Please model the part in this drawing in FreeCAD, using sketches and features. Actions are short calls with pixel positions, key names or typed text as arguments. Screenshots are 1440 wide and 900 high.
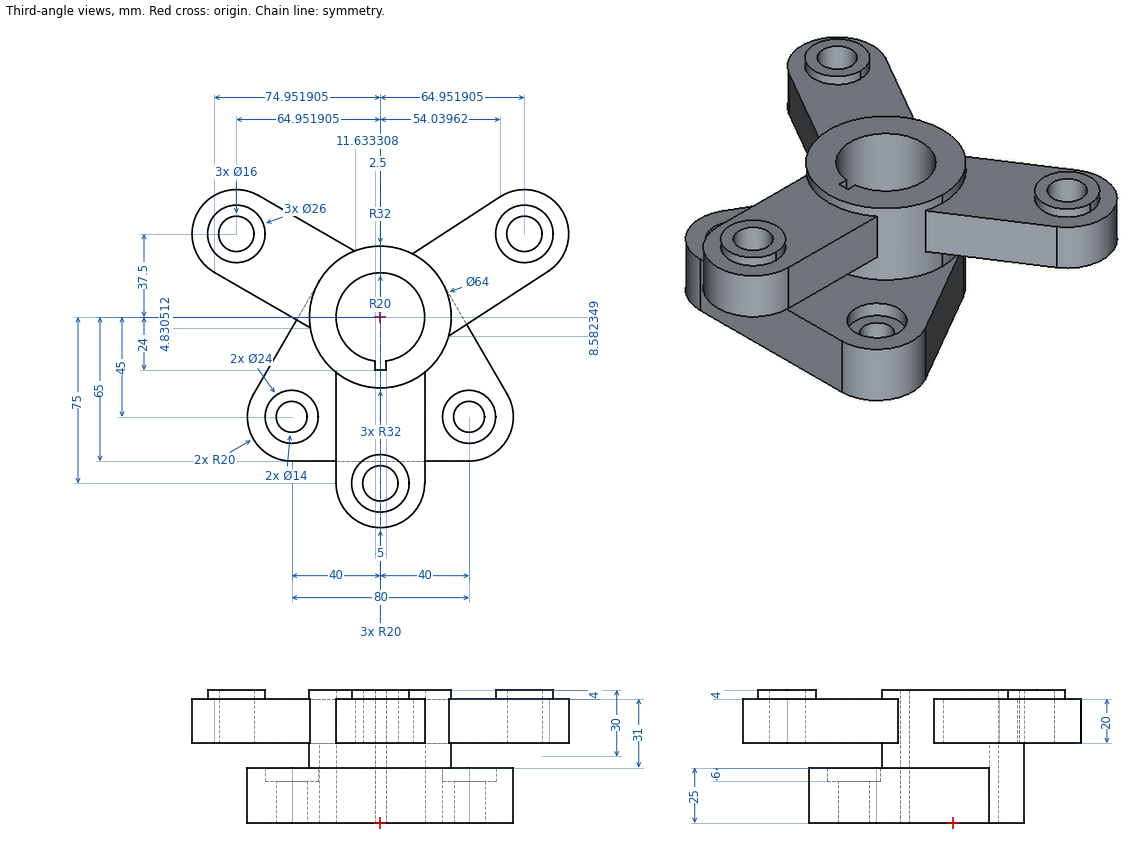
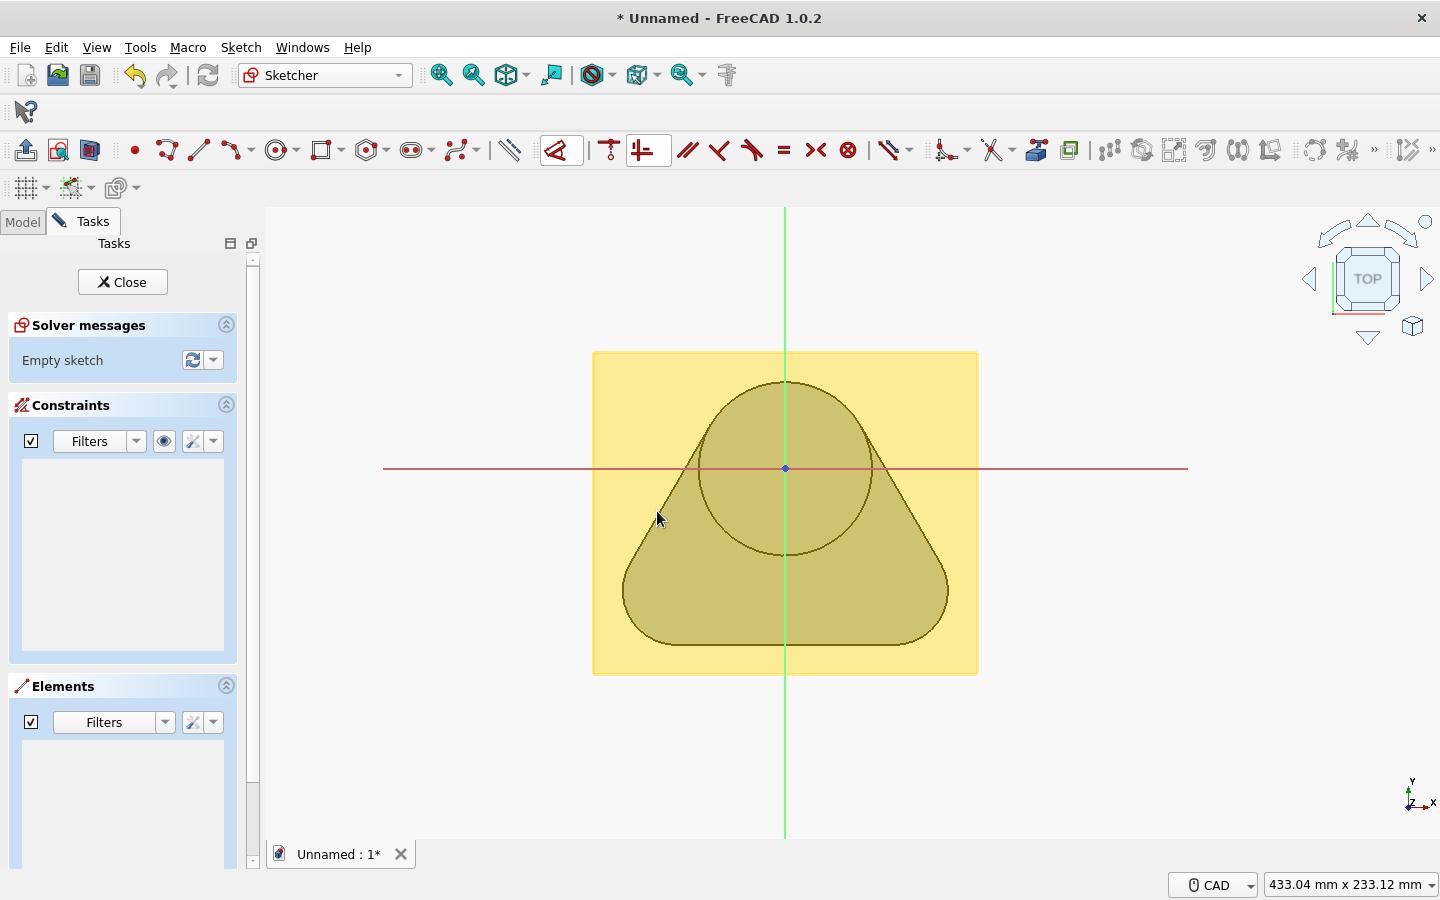
click(200, 150)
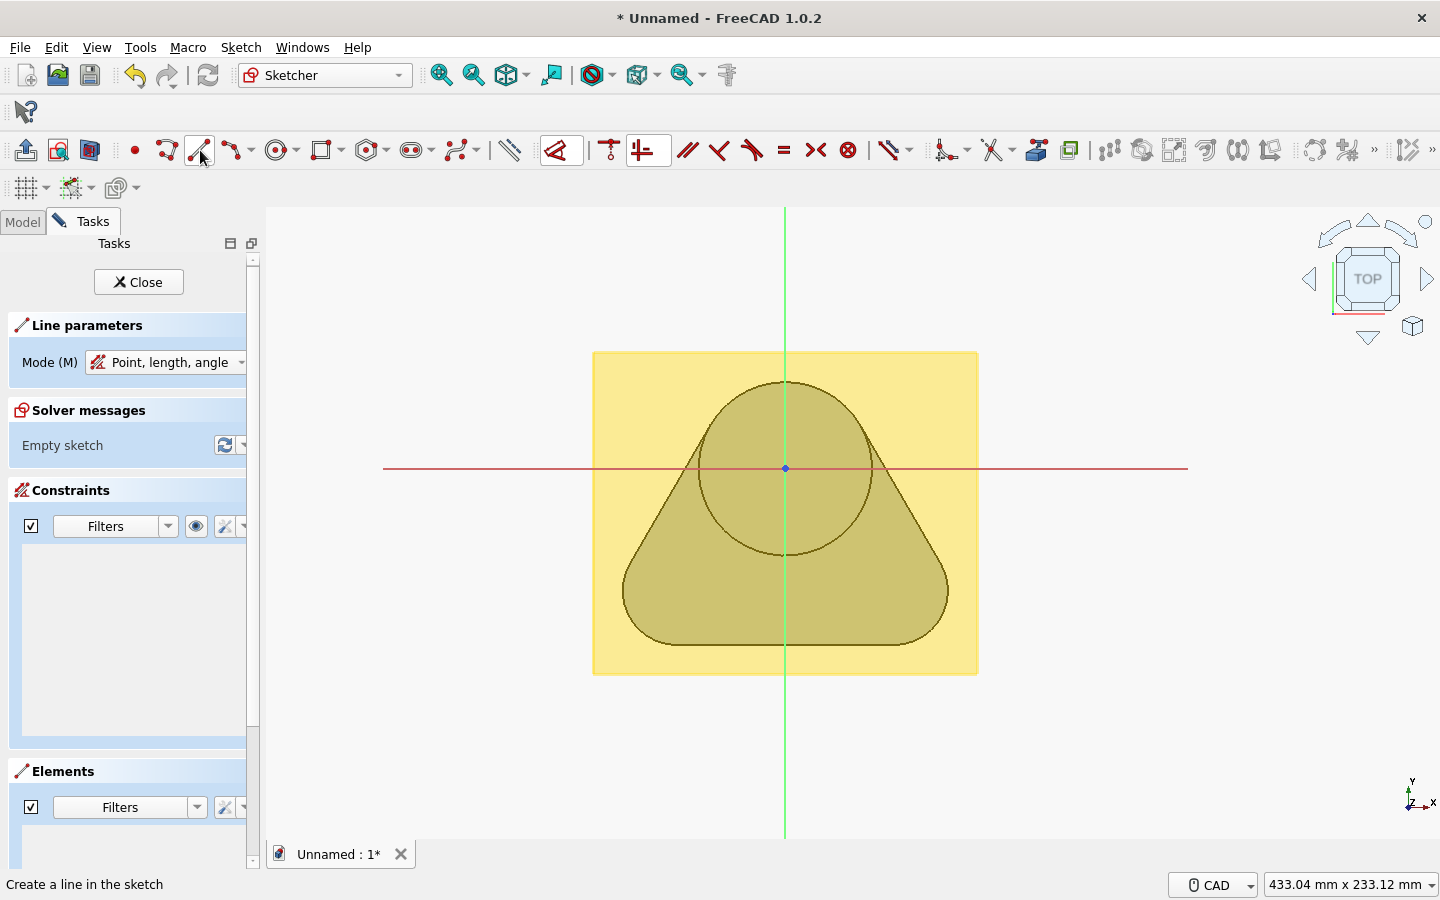
click(731, 537)
click(731, 672)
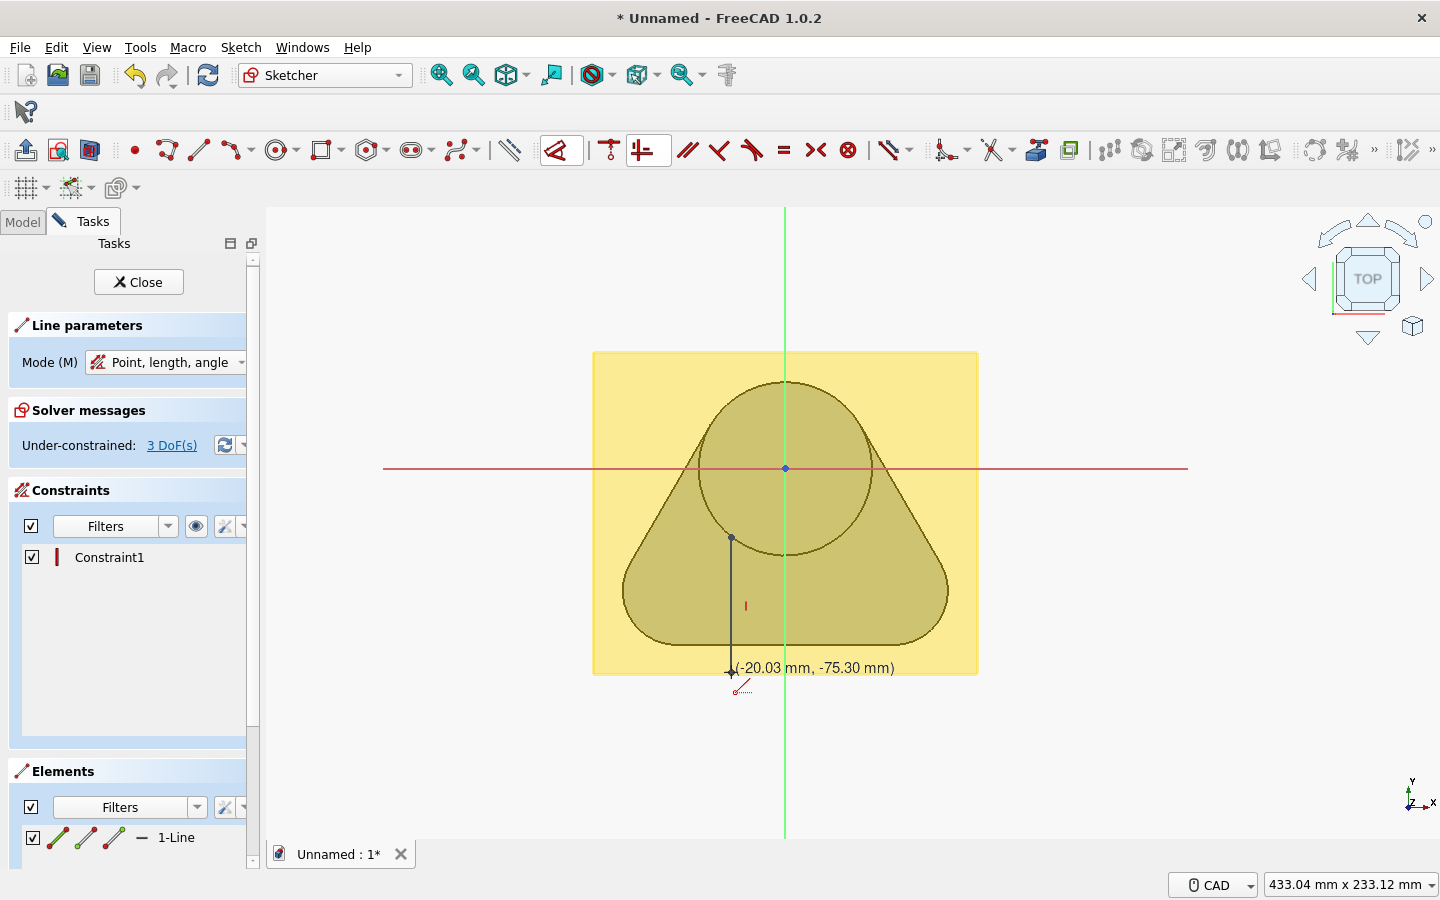
click(840, 672)
click(840, 537)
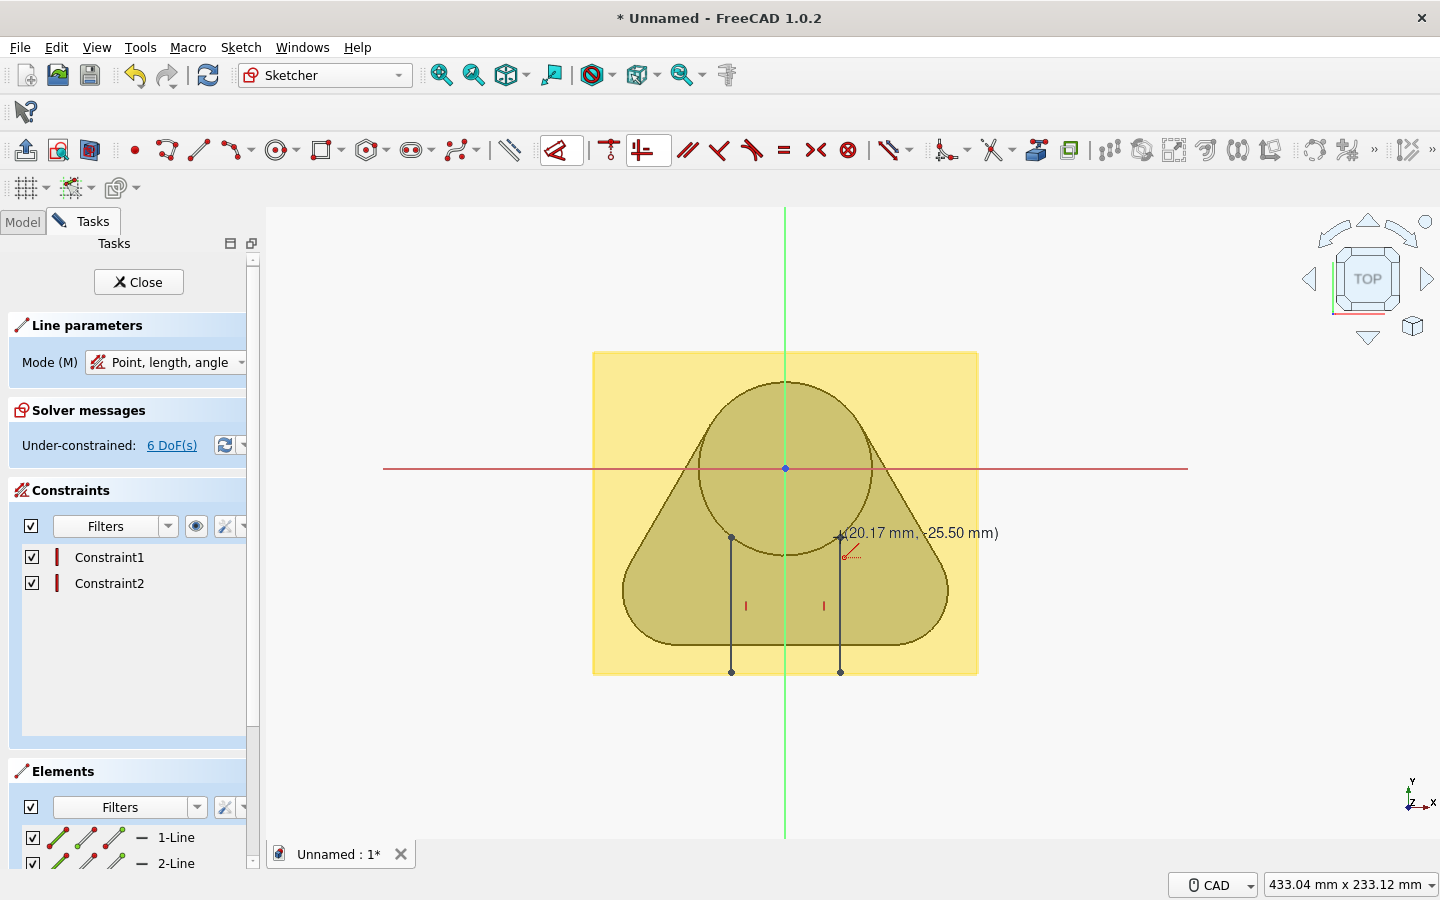
click(232, 150)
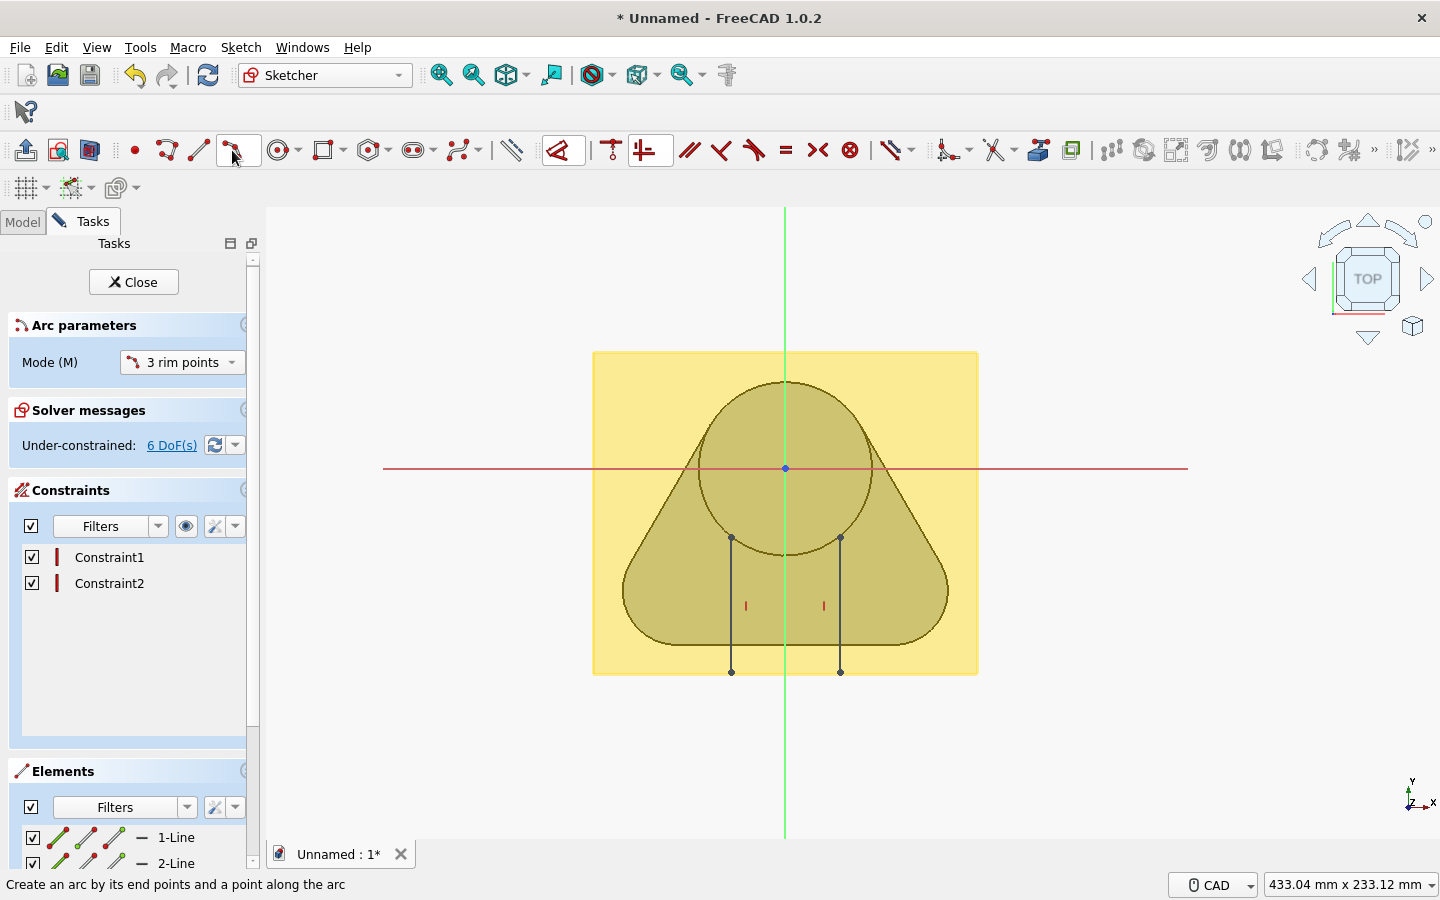
click(731, 673)
click(840, 673)
click(769, 724)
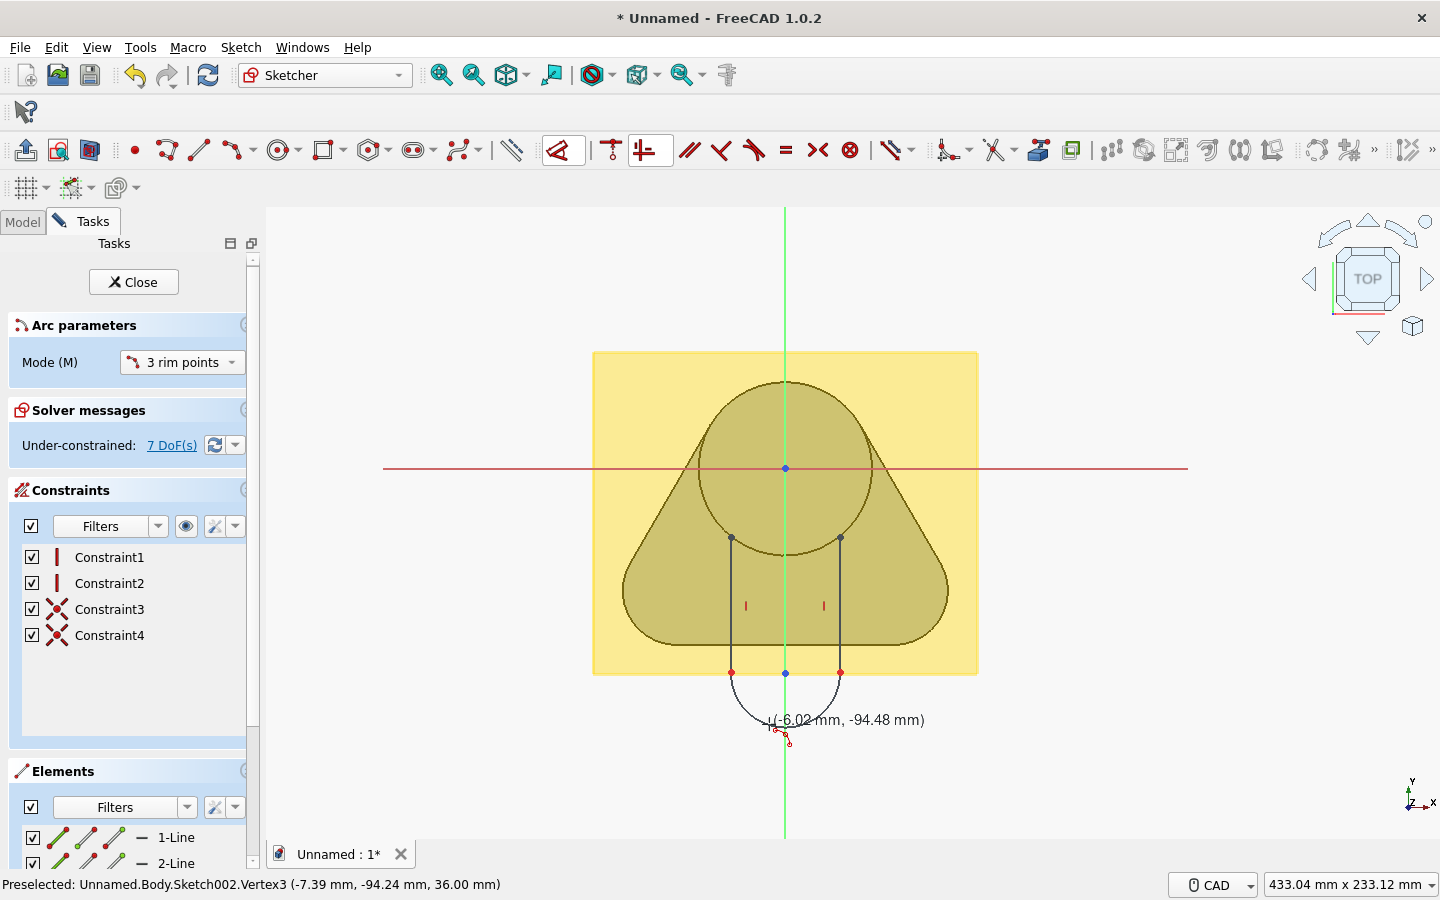
click(840, 538)
click(731, 538)
click(762, 552)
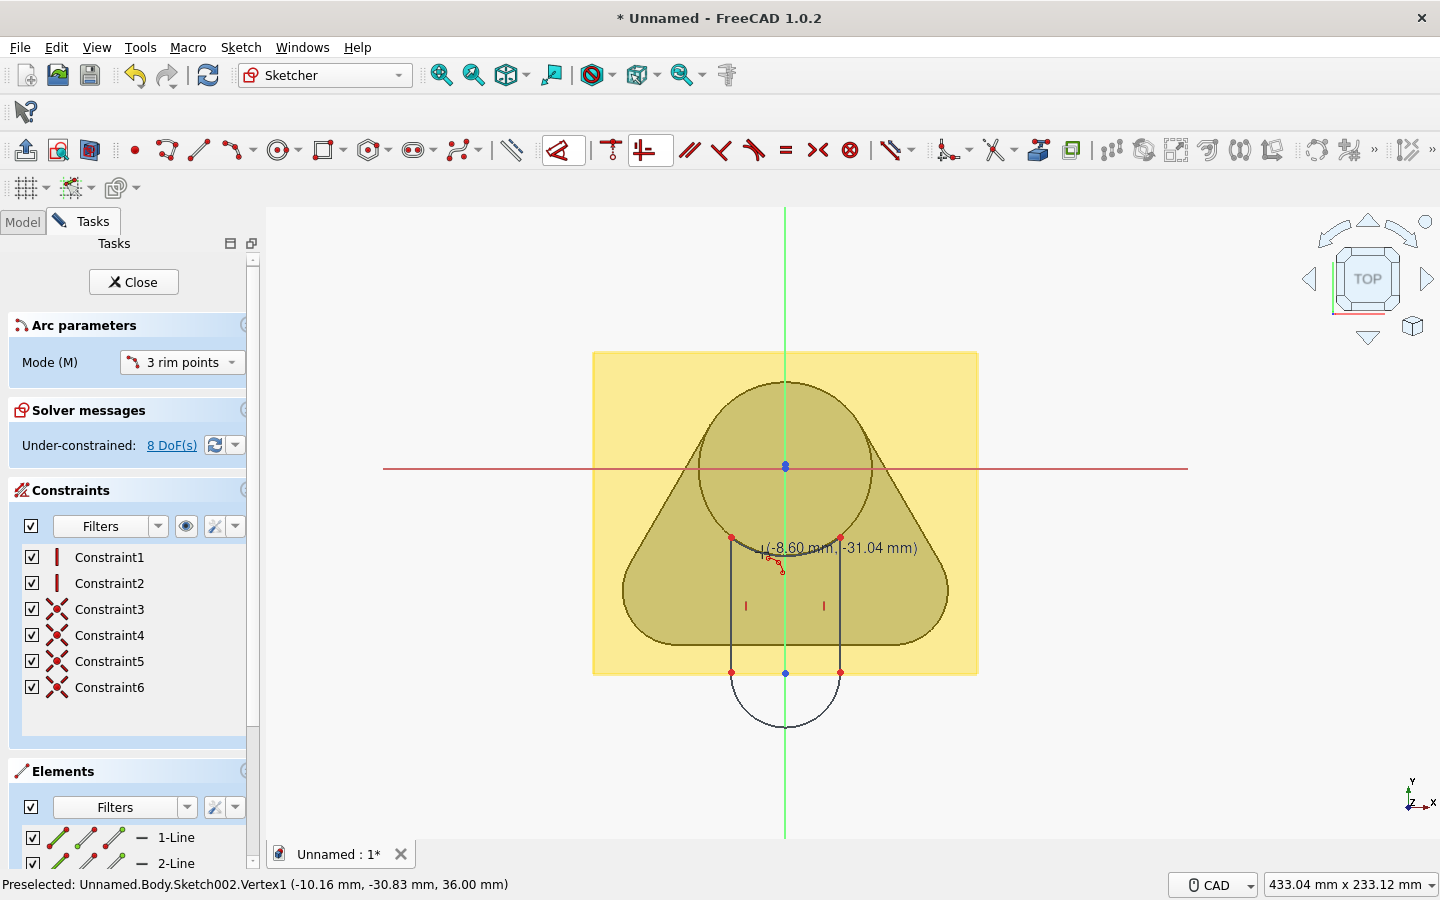
click(200, 150)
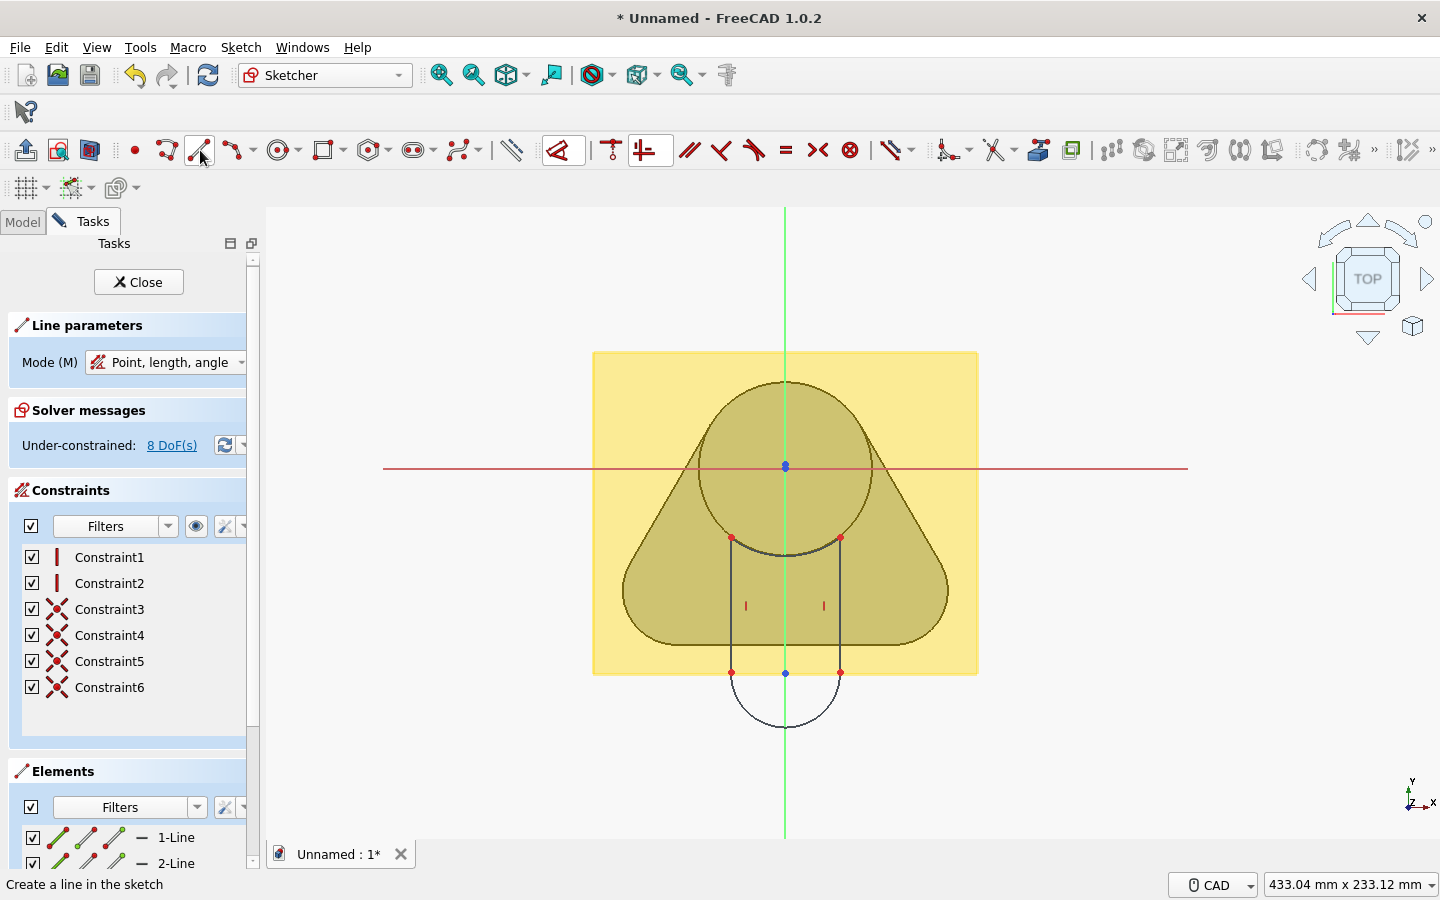
click(582, 414)
click(700, 482)